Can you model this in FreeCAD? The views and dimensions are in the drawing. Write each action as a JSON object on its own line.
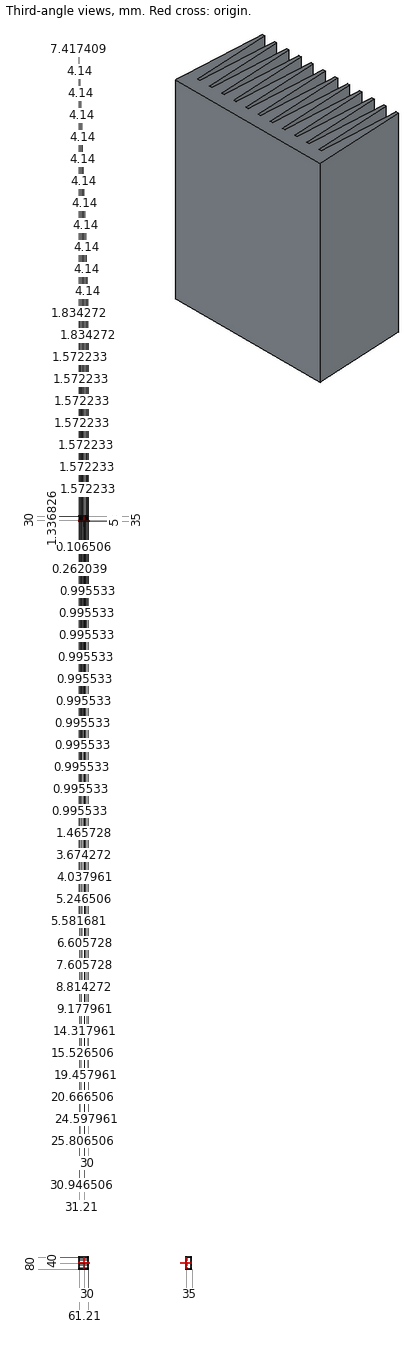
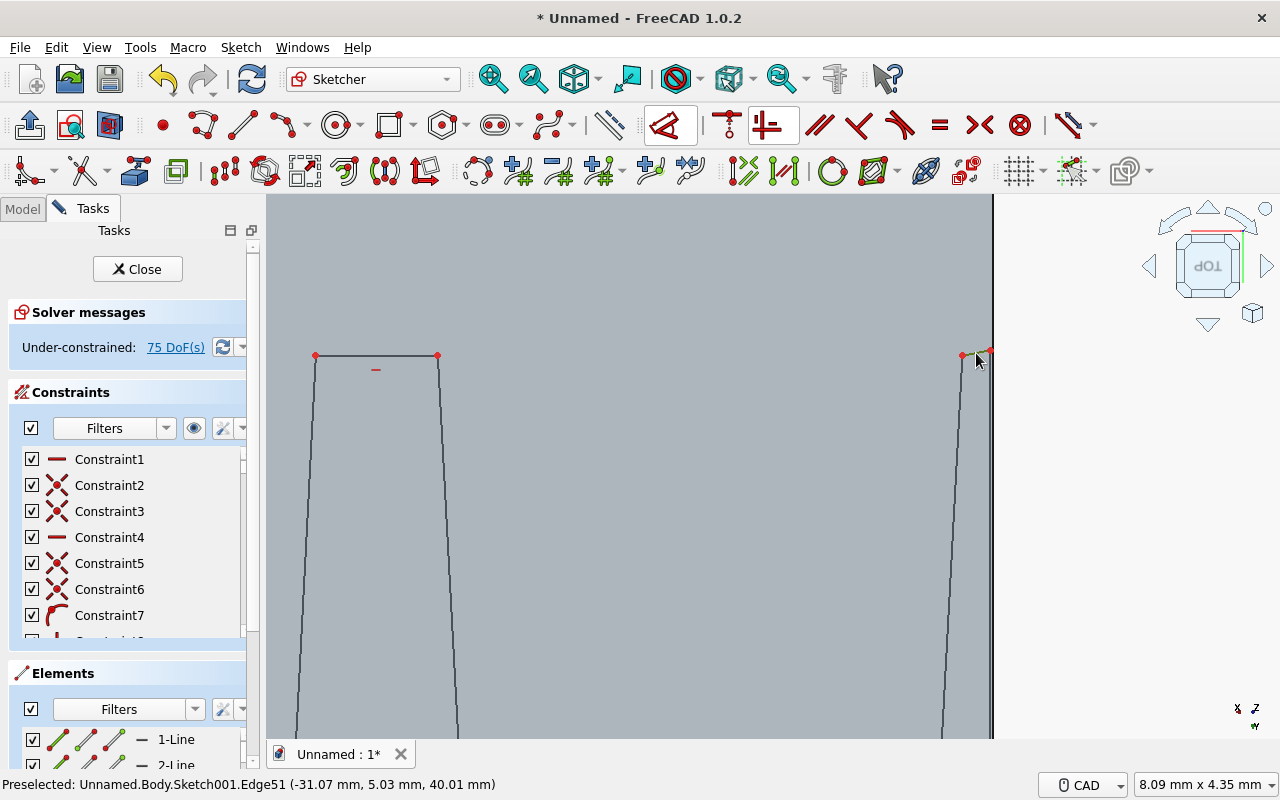
{"action": "key", "text": "h"}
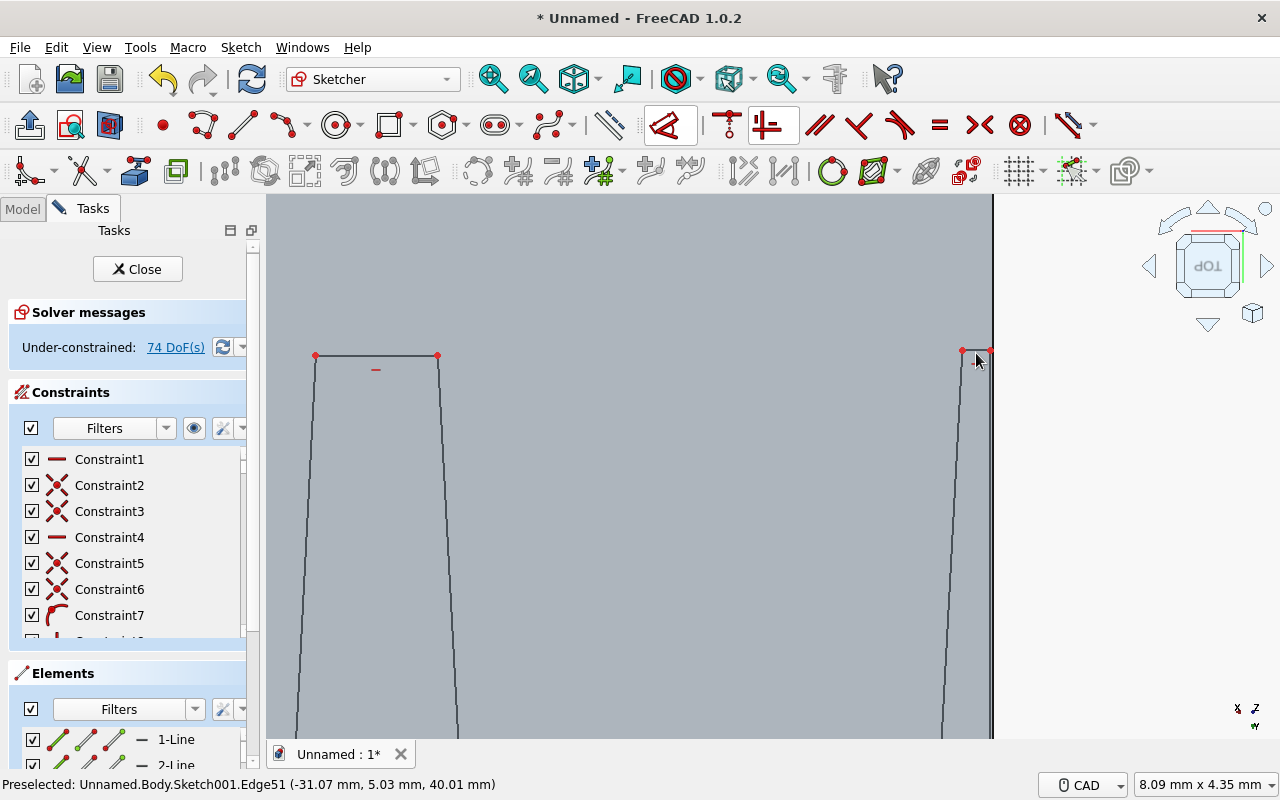
{"action": "scroll", "coordinate": [989, 350], "scroll_direction": "down", "scroll_amount": 13}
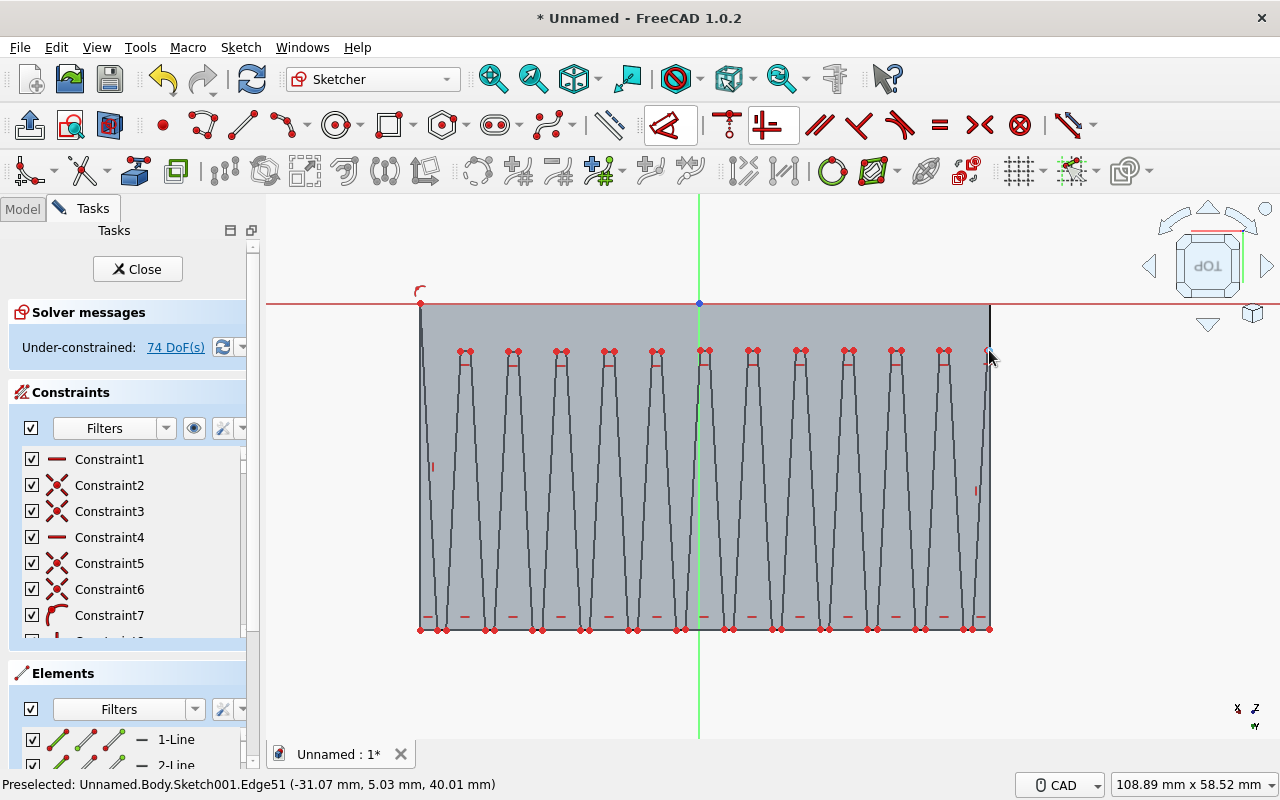
{"action": "scroll", "coordinate": [420, 402], "scroll_direction": "up", "scroll_amount": 5}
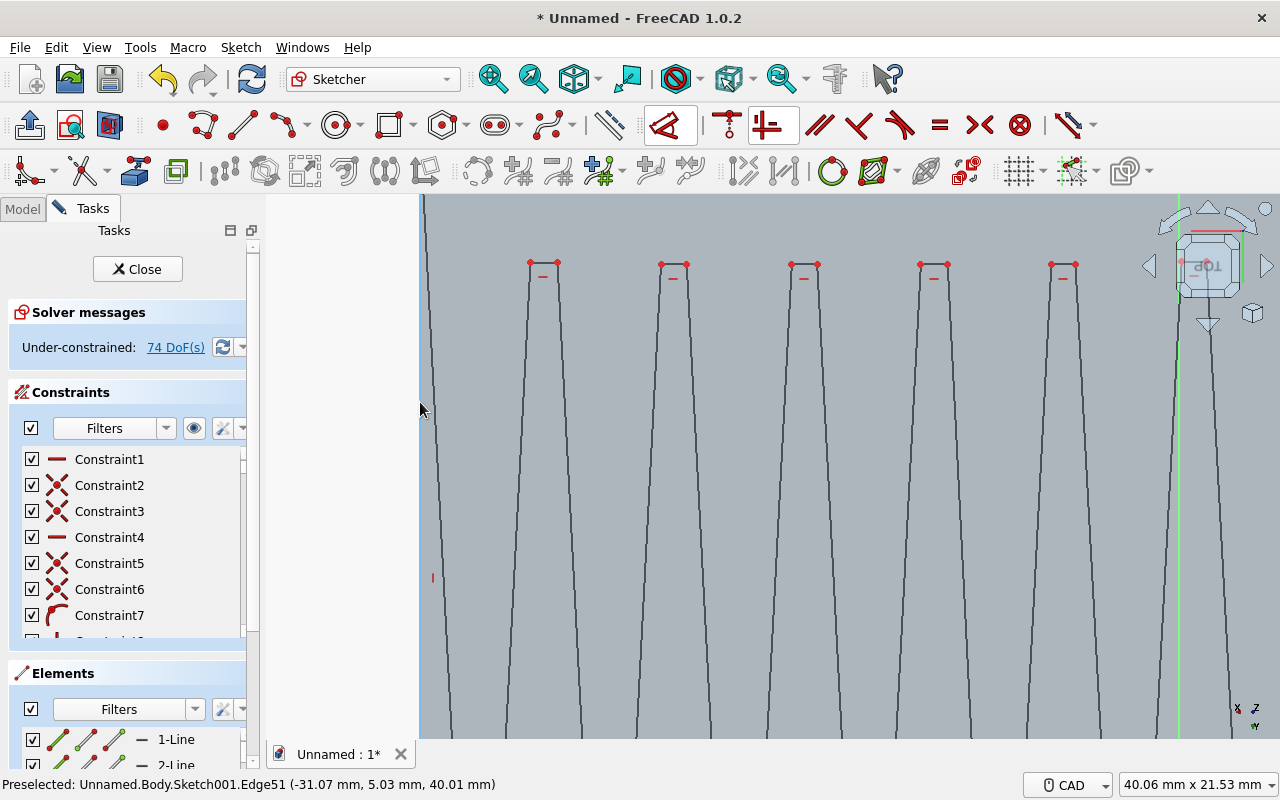
{"action": "left_click", "coordinate": [420, 400]}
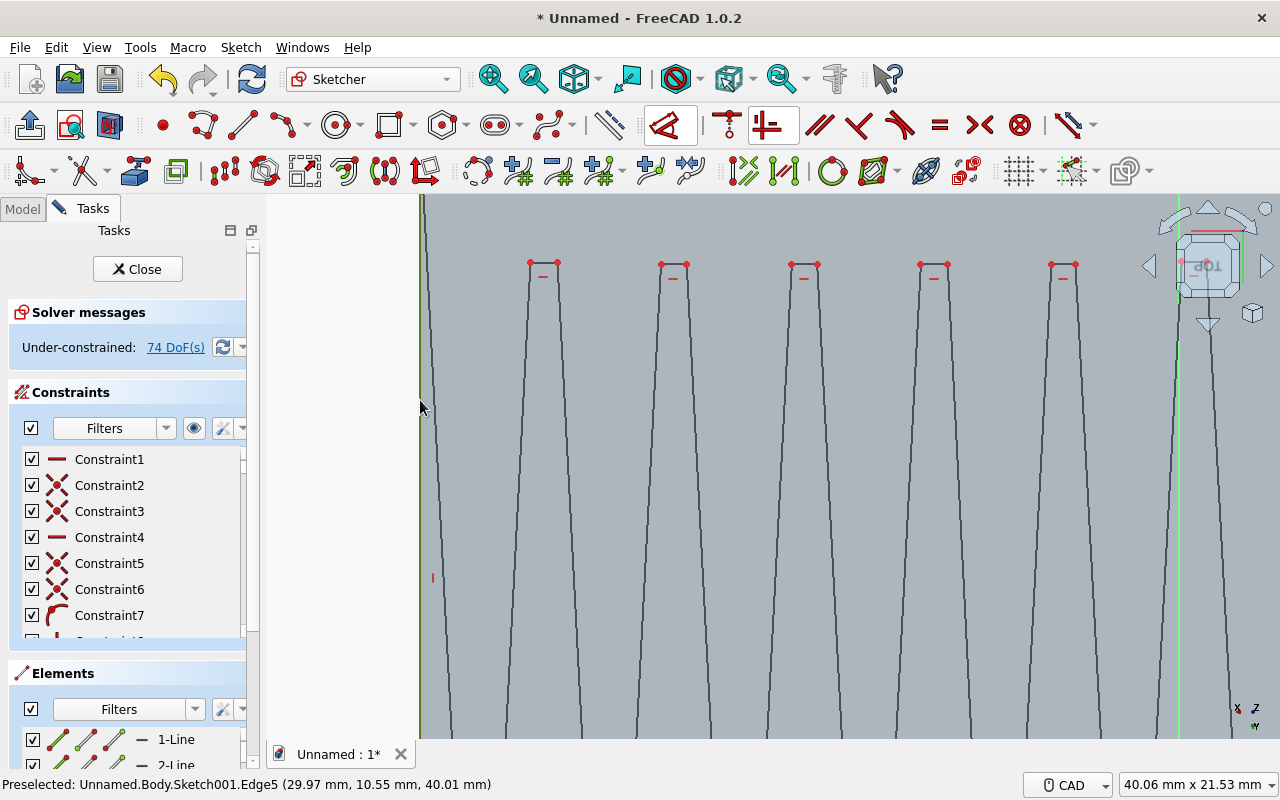
{"action": "left_click", "coordinate": [692, 126]}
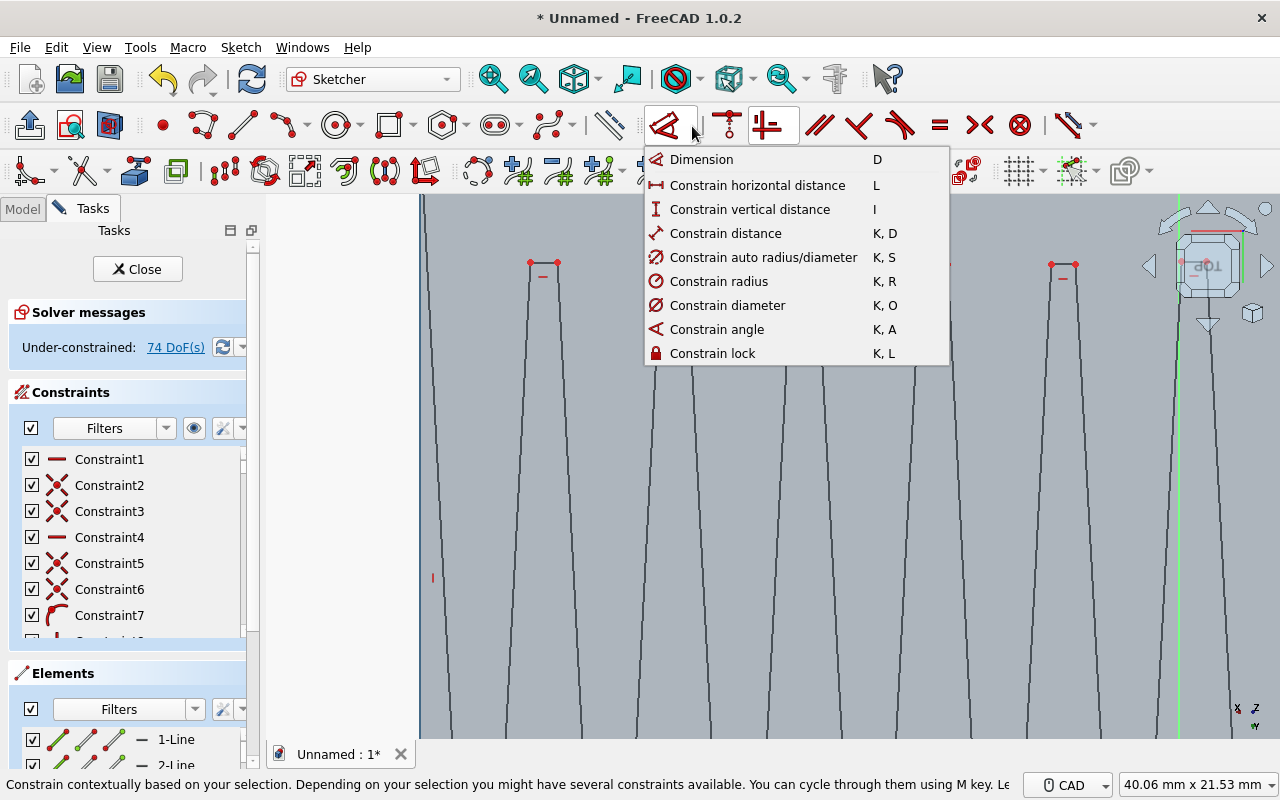
{"action": "left_click", "coordinate": [797, 209]}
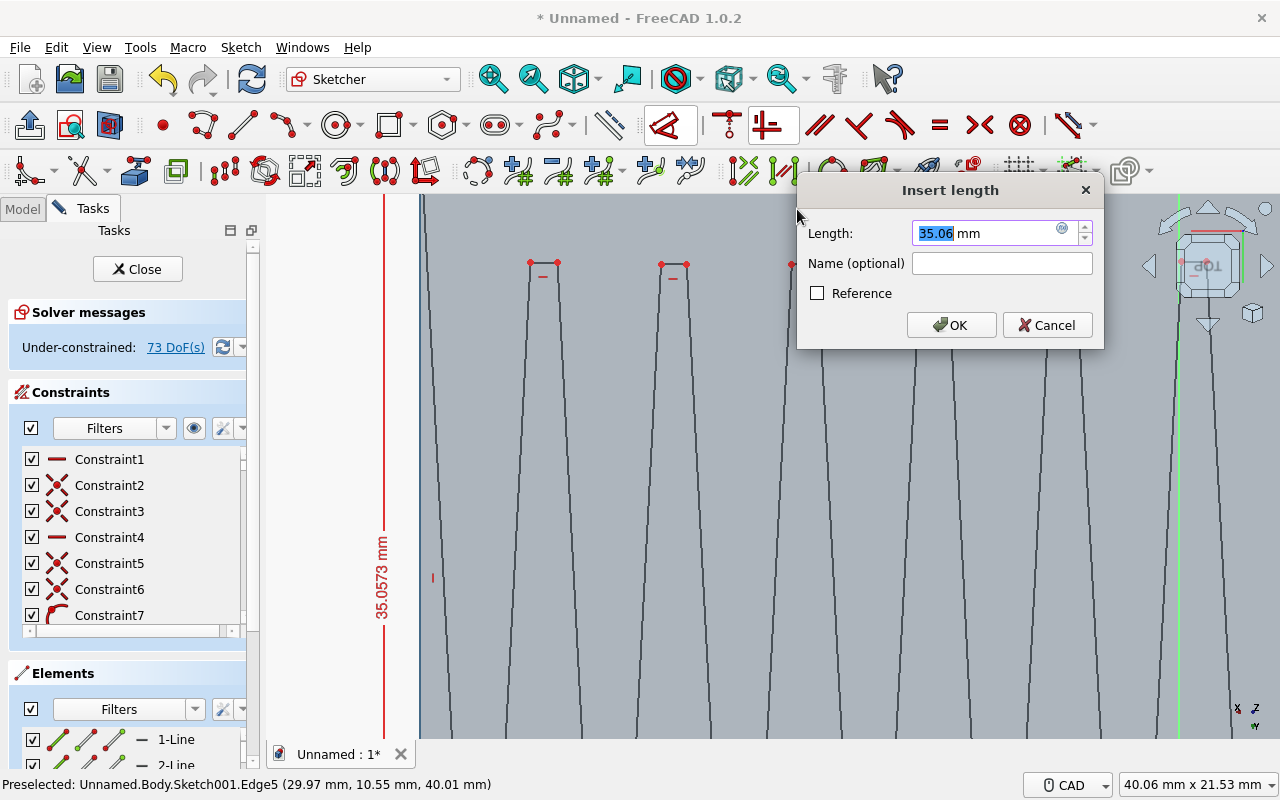
{"action": "type", "text": "35"}
{"action": "key", "text": "Return"}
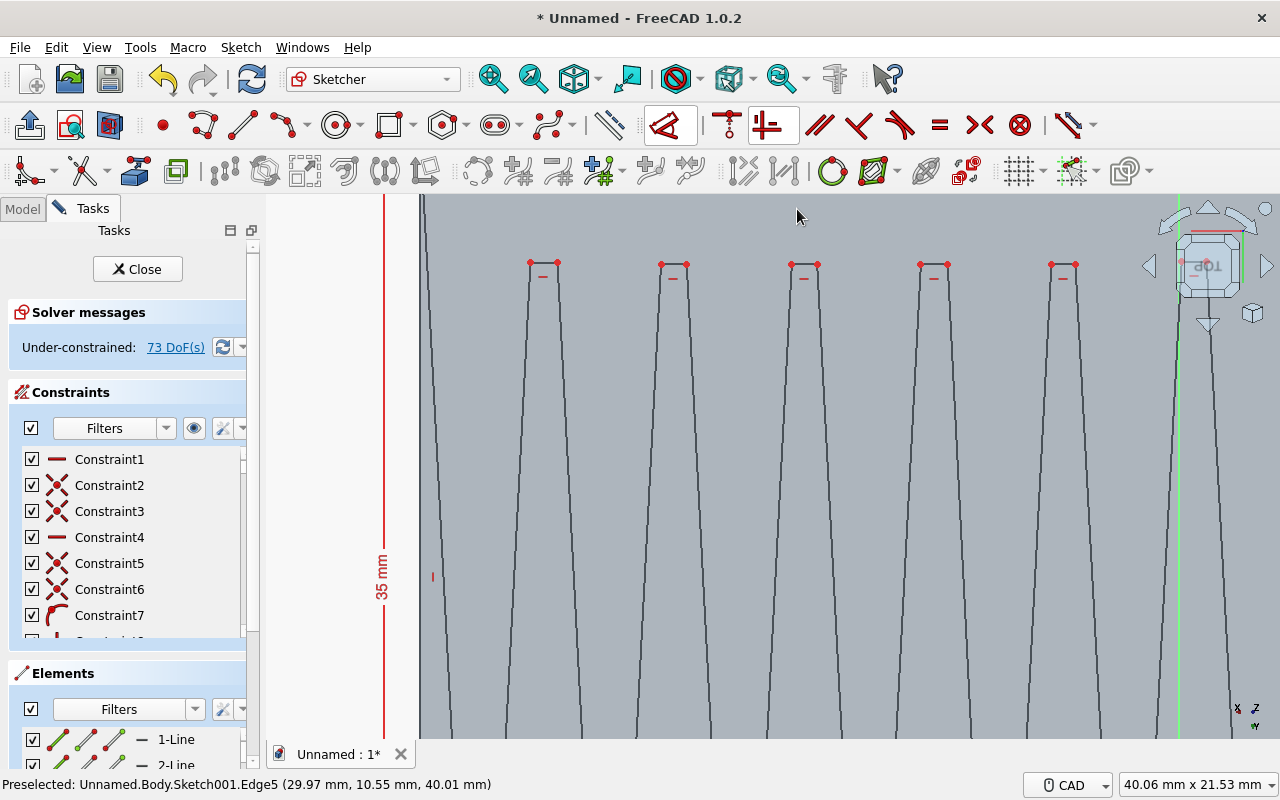
{"action": "scroll", "coordinate": [419, 402], "scroll_direction": "down", "scroll_amount": 5}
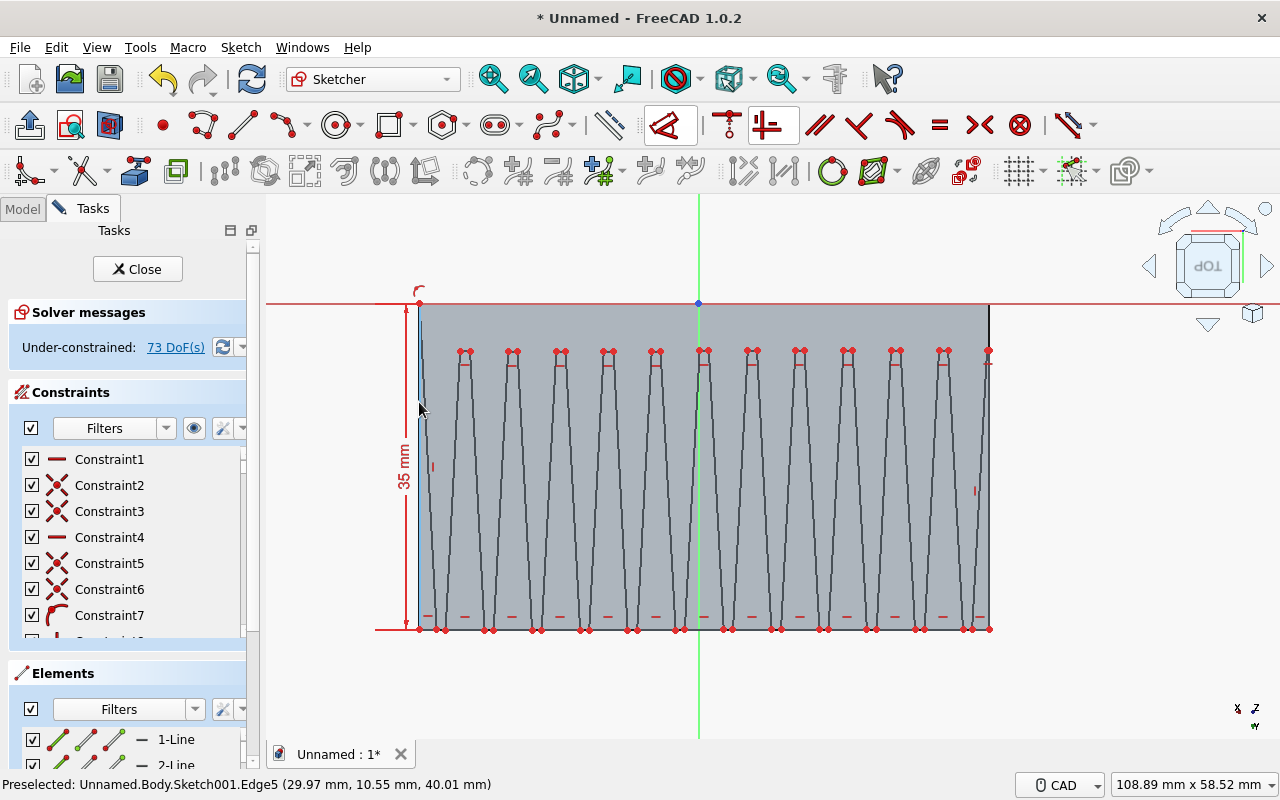
{"action": "left_click", "coordinate": [989, 546]}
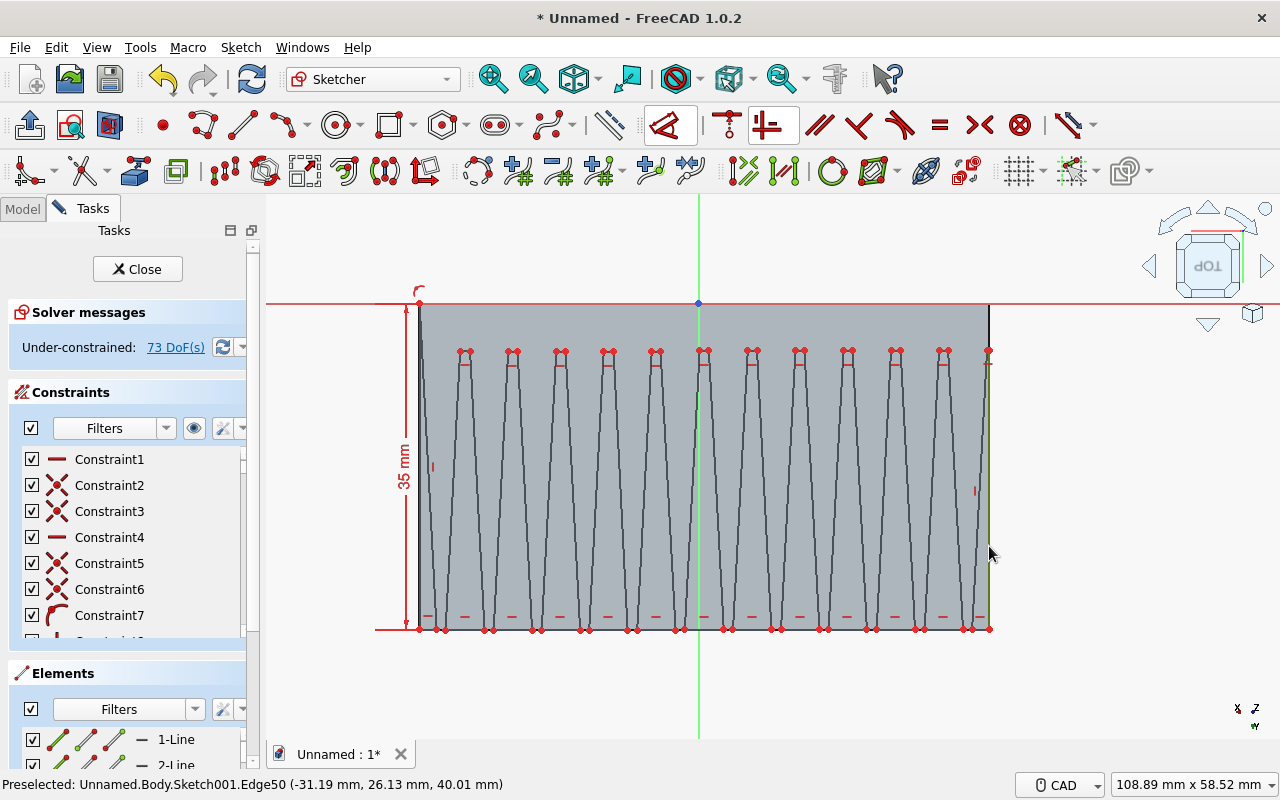
{"action": "key", "text": "i"}